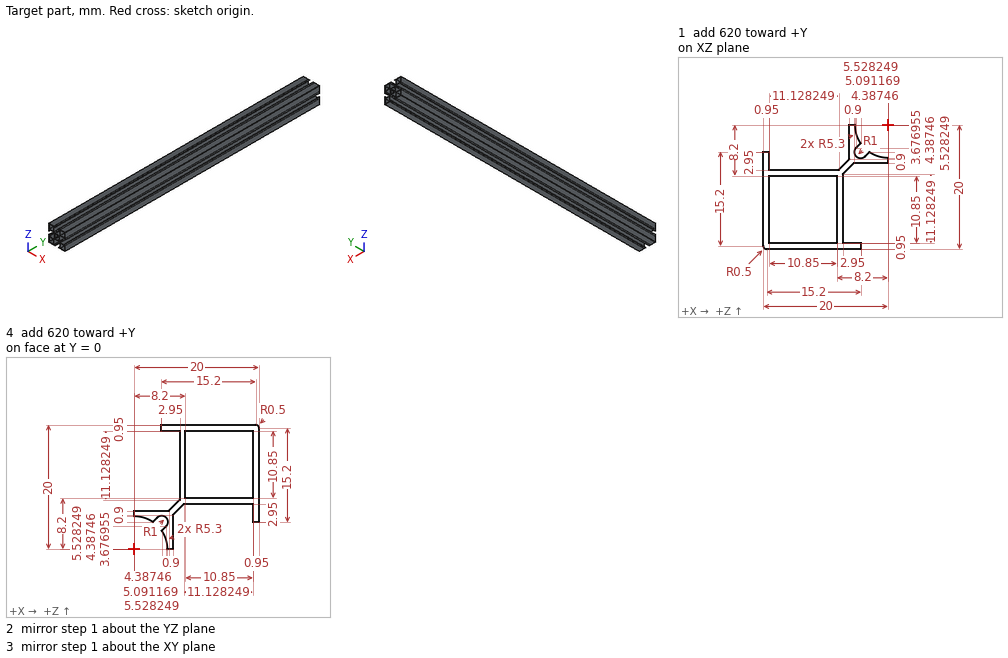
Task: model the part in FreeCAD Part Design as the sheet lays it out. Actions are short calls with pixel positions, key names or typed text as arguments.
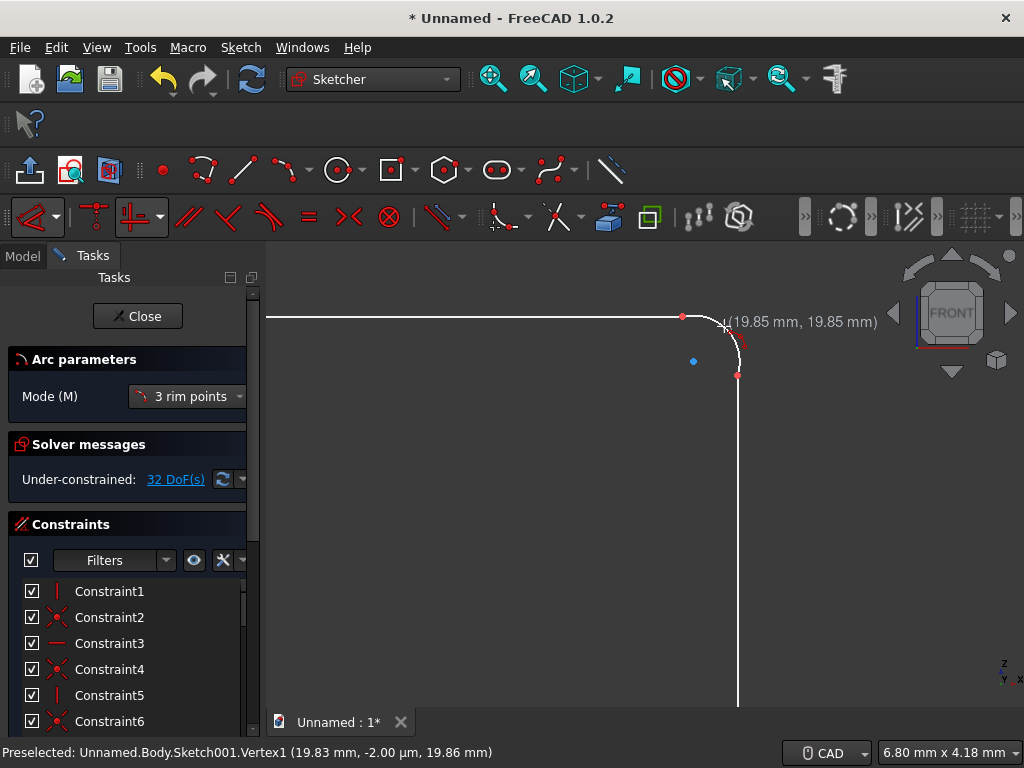
click(418, 170)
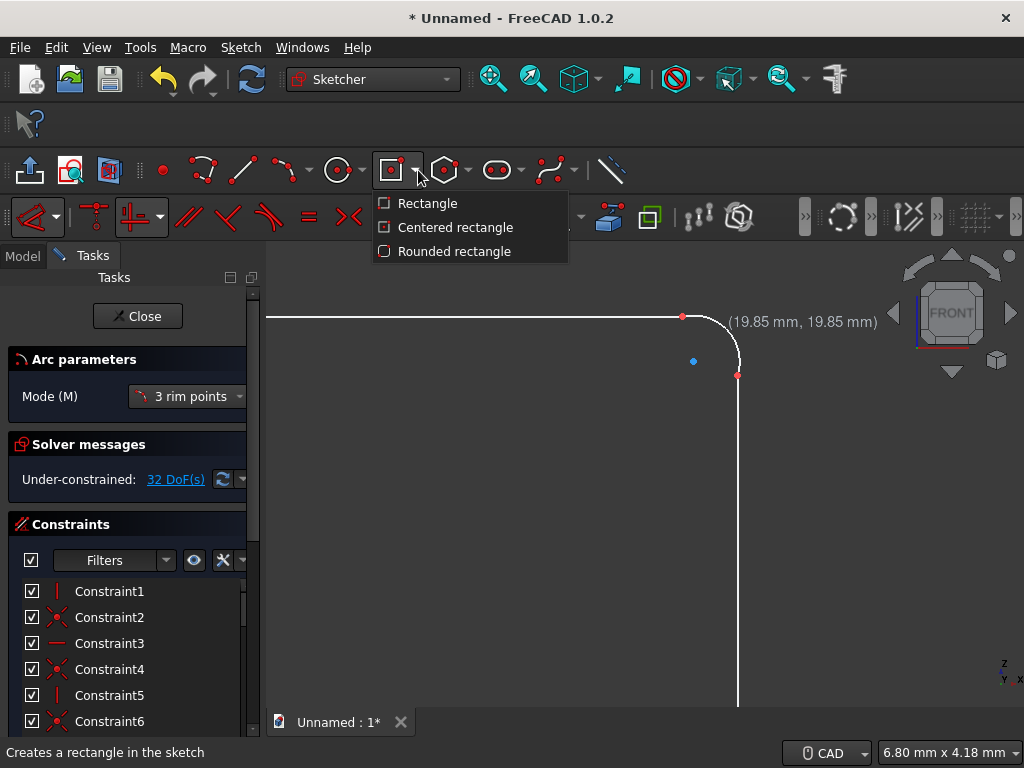
click(470, 203)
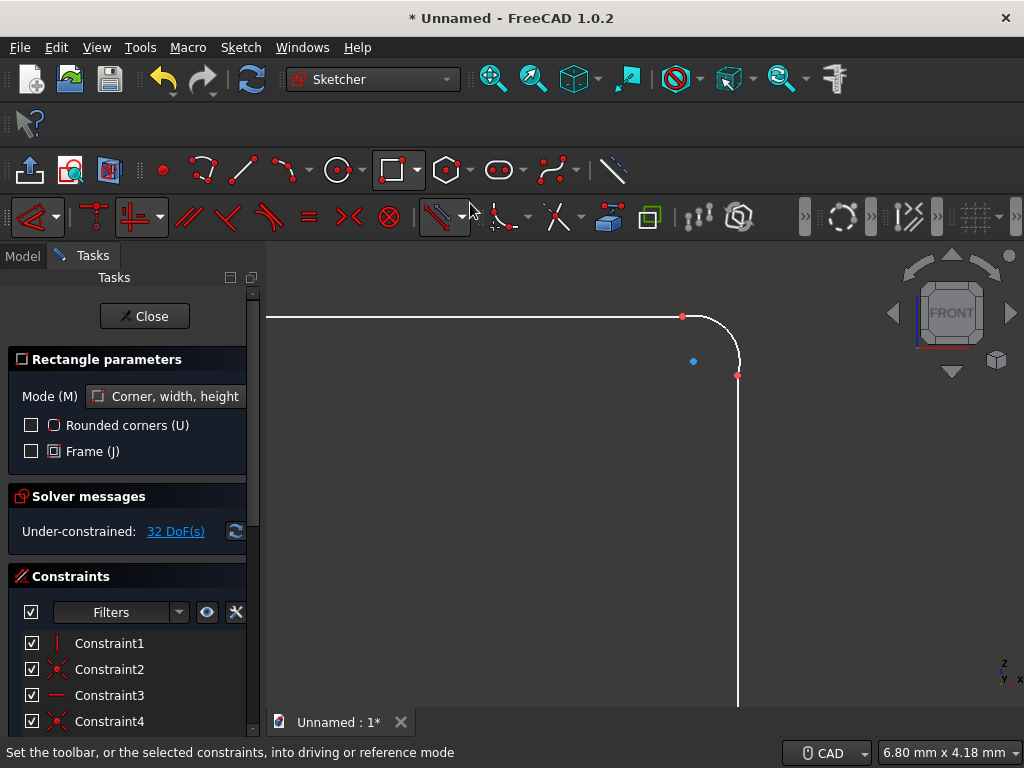
scroll(725, 325, down, 10)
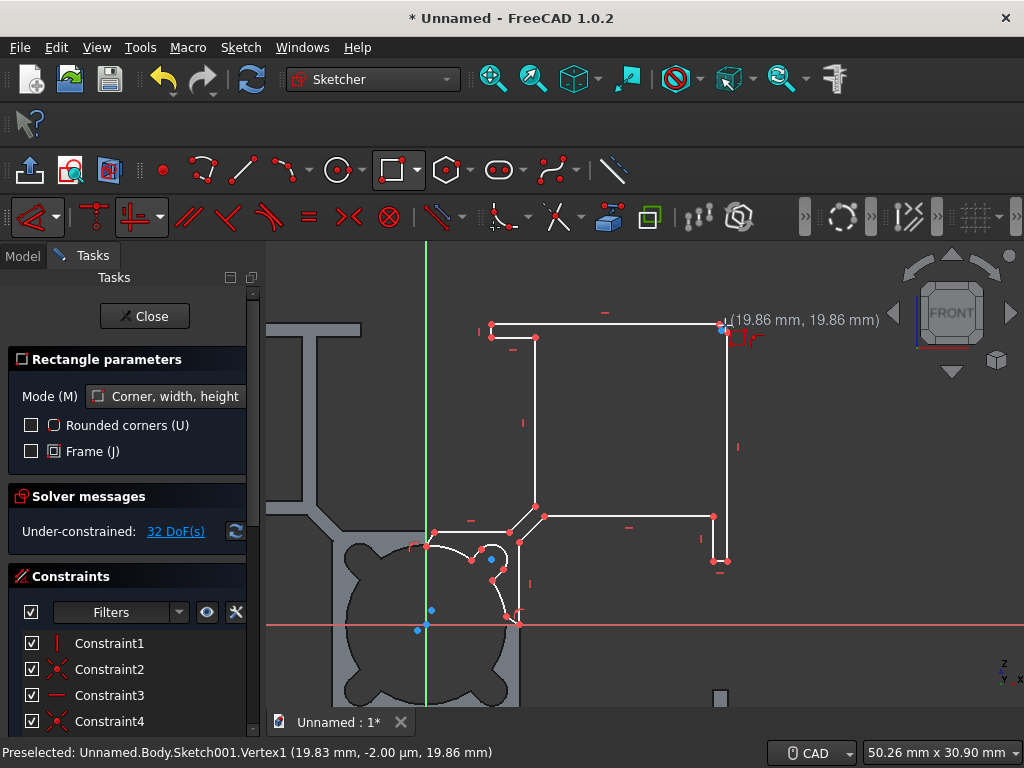
click(550, 337)
move(713, 501)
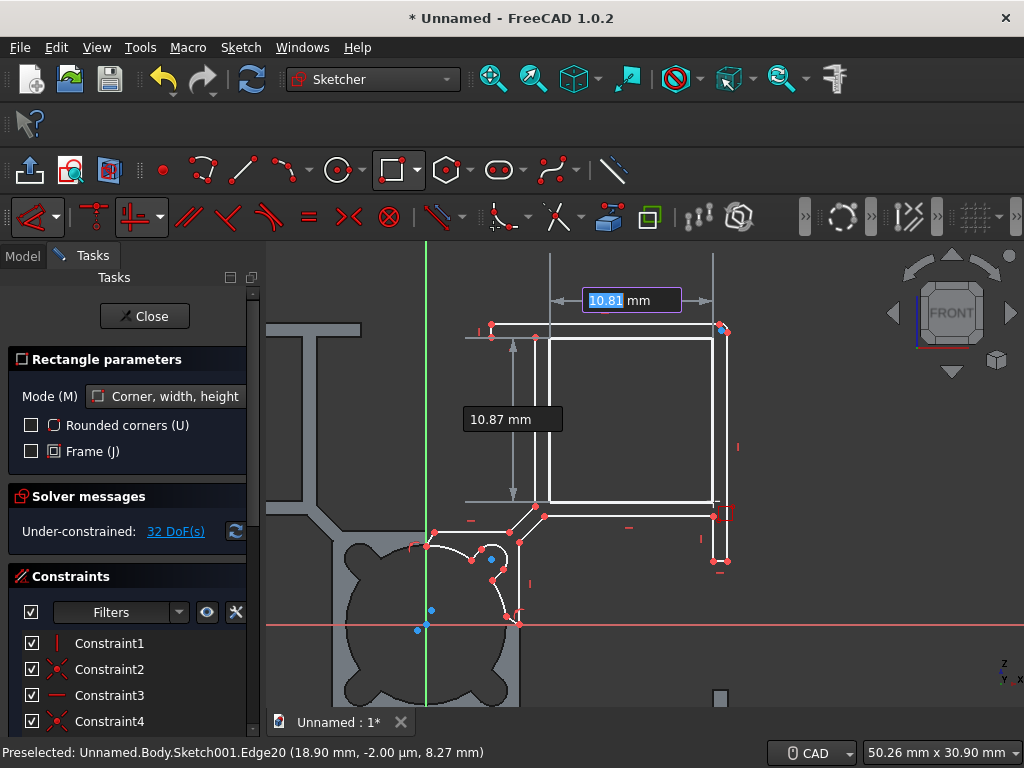
text(10.85)
key(Tab)
text(10.85)
key(Return)
key(Escape)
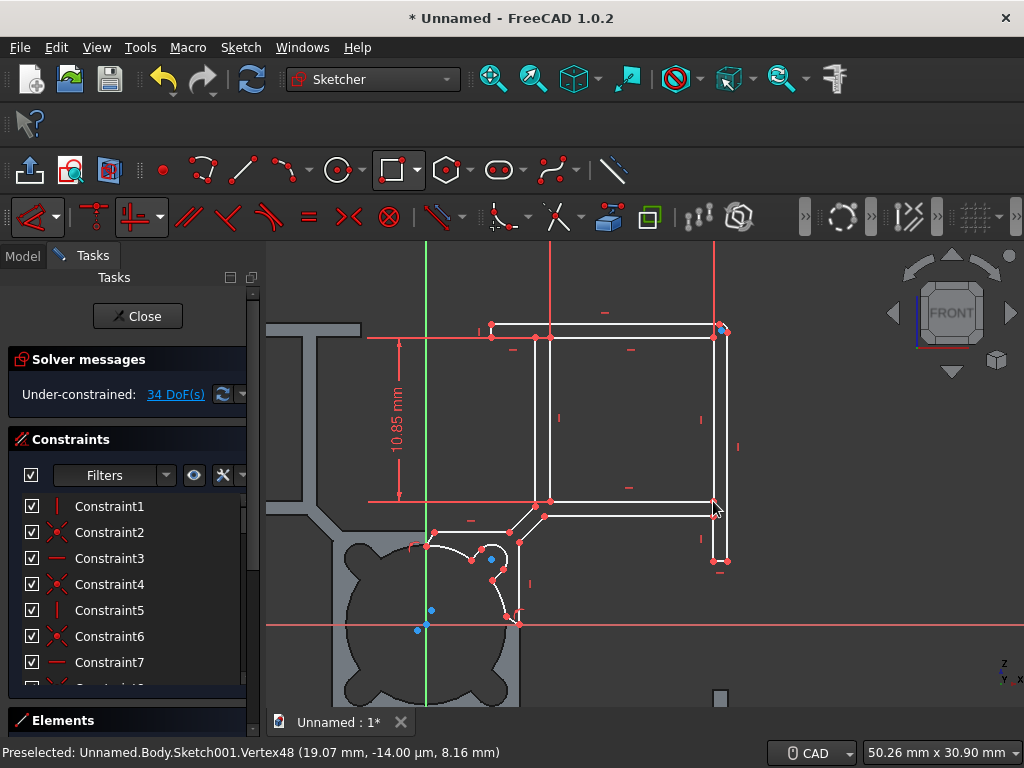
click(727, 401)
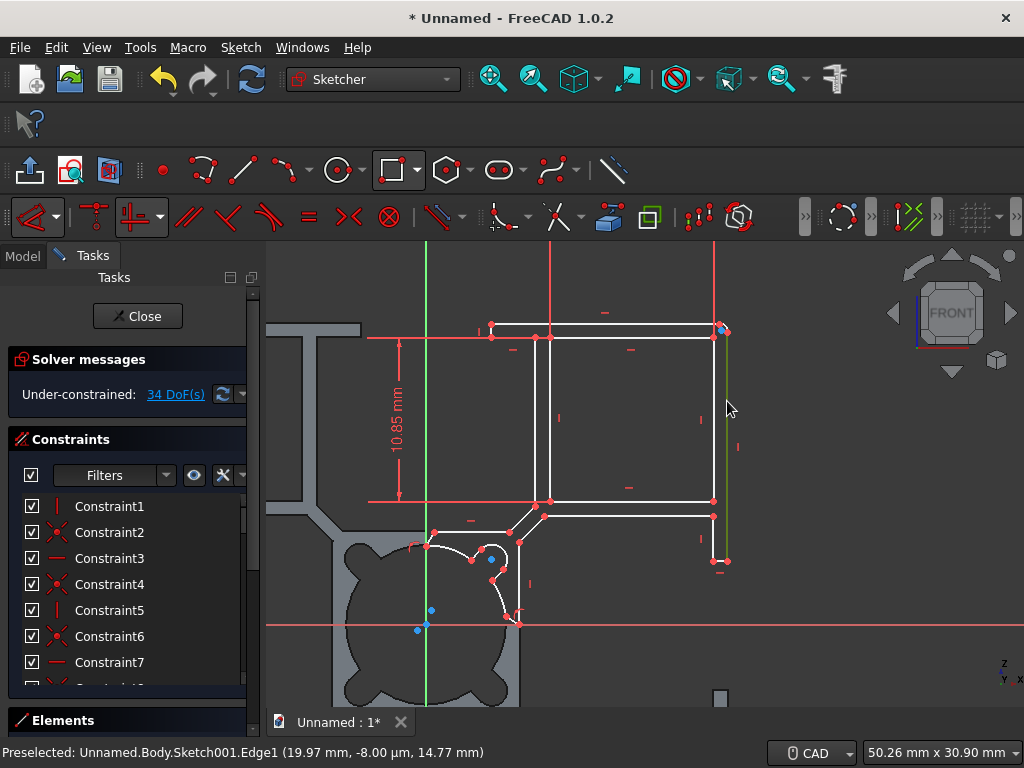
scroll(726, 326, up, 4)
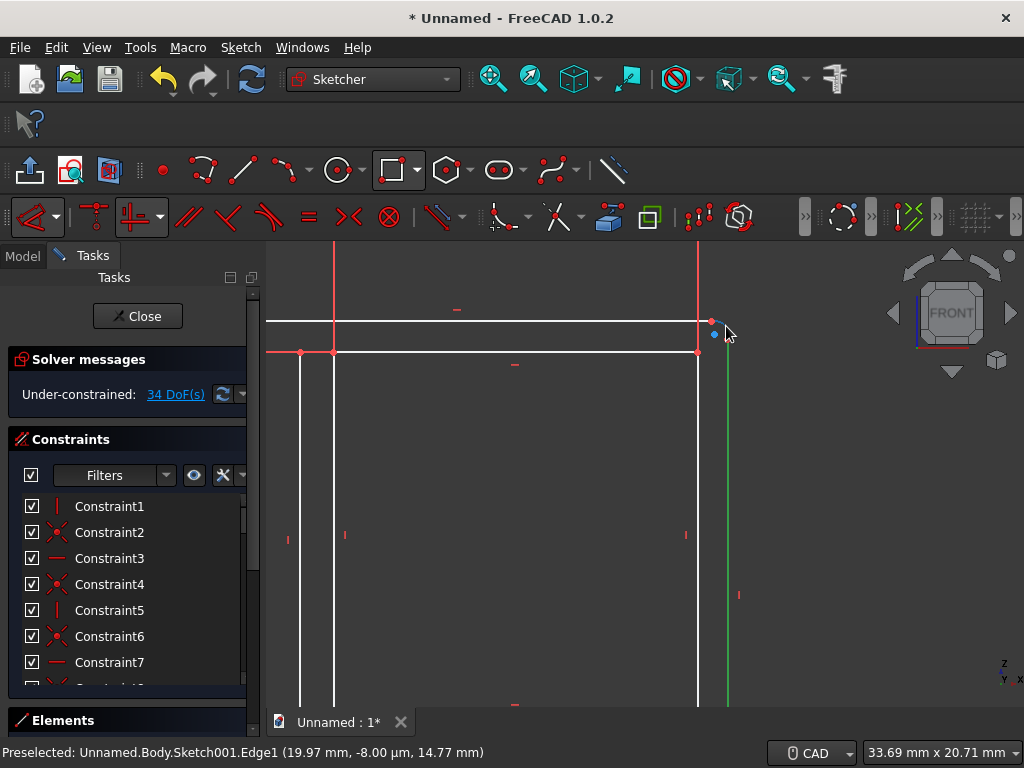
click(725, 325)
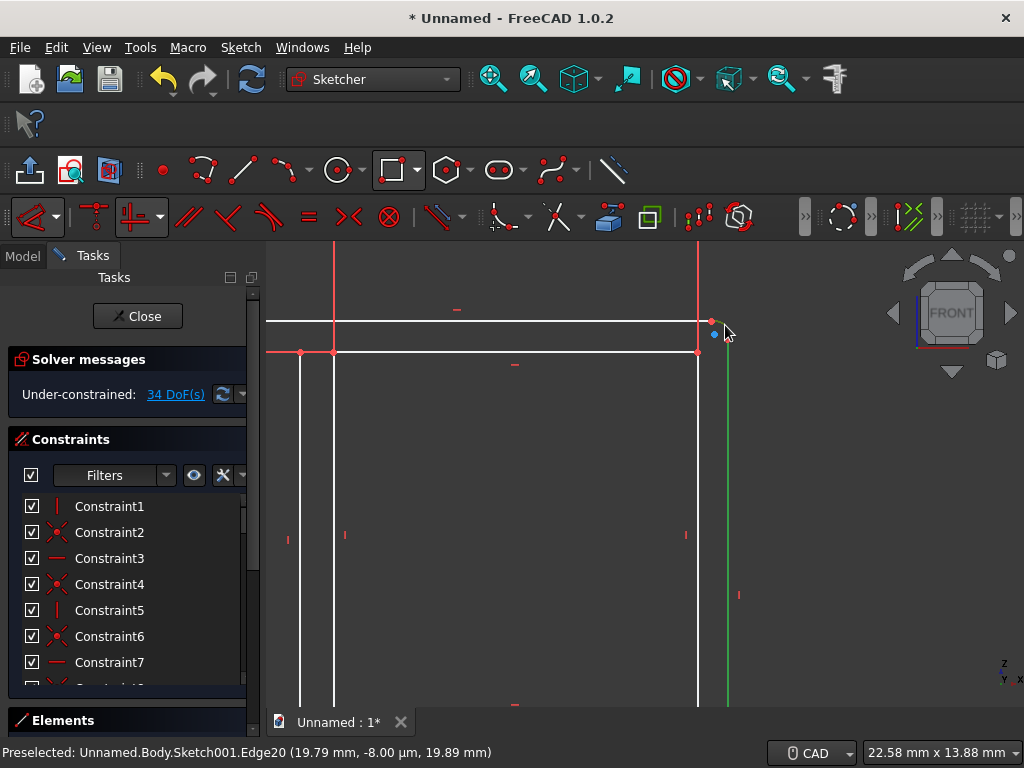
click(270, 218)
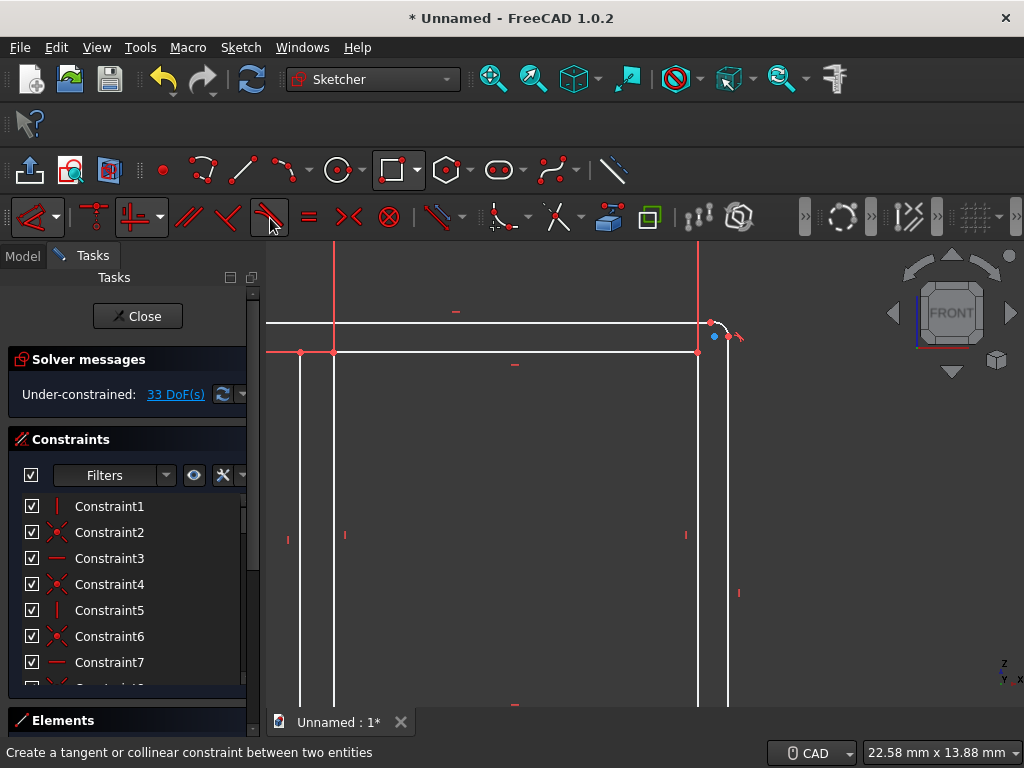
scroll(726, 326, down, 4)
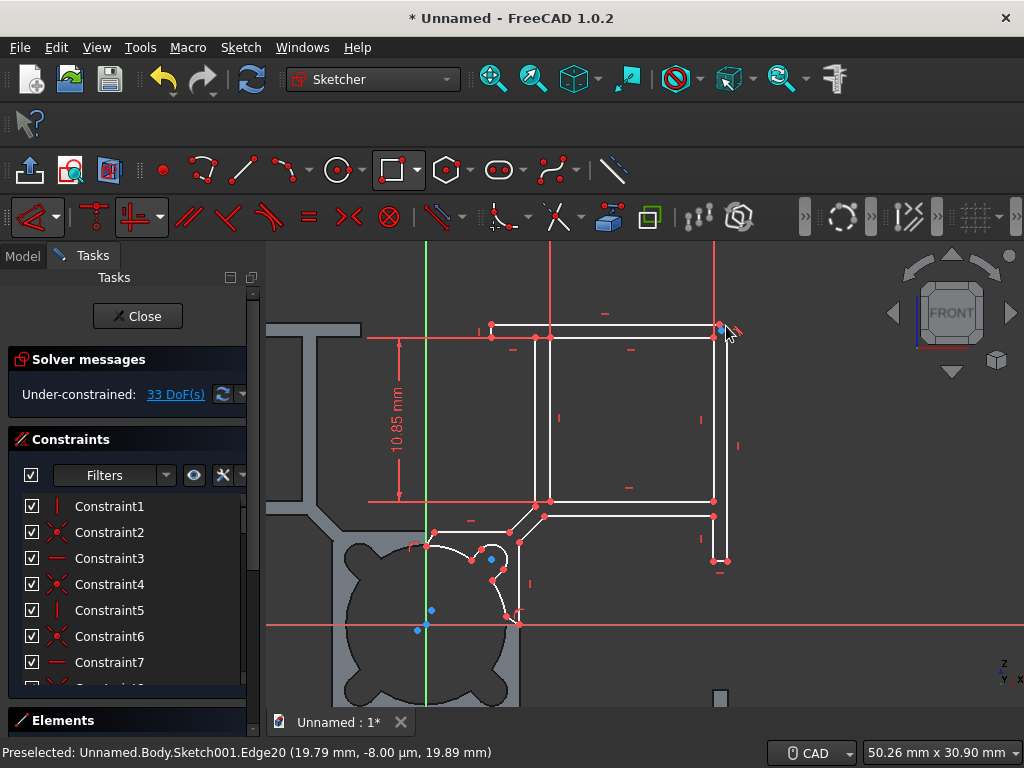
scroll(496, 578, up, 6)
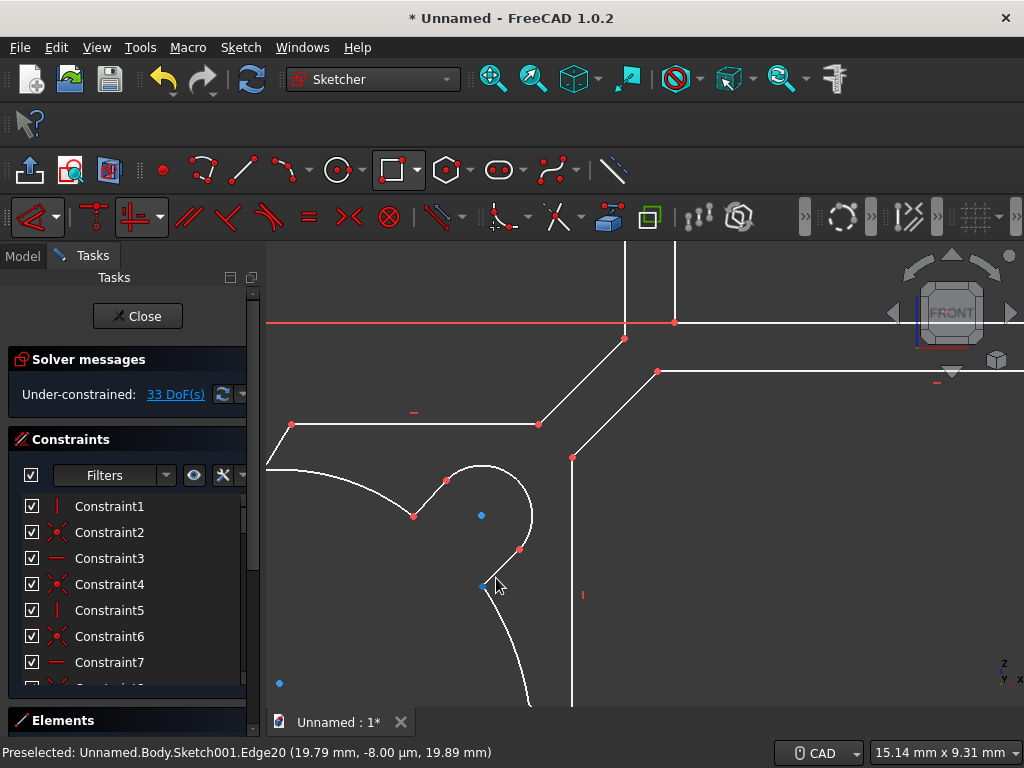
click(494, 575)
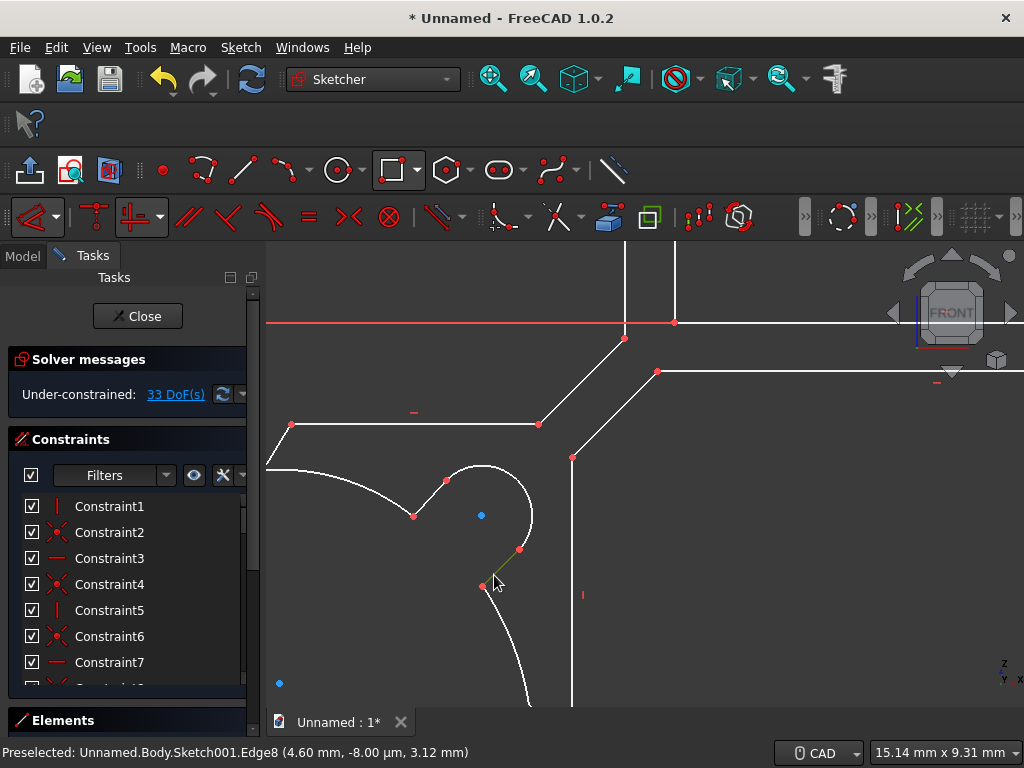
click(531, 506)